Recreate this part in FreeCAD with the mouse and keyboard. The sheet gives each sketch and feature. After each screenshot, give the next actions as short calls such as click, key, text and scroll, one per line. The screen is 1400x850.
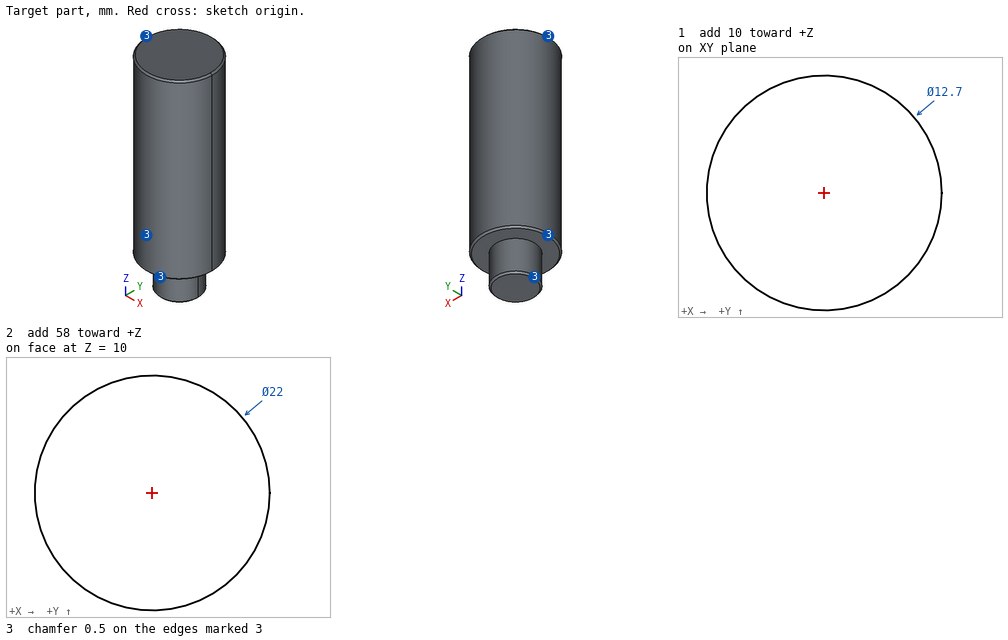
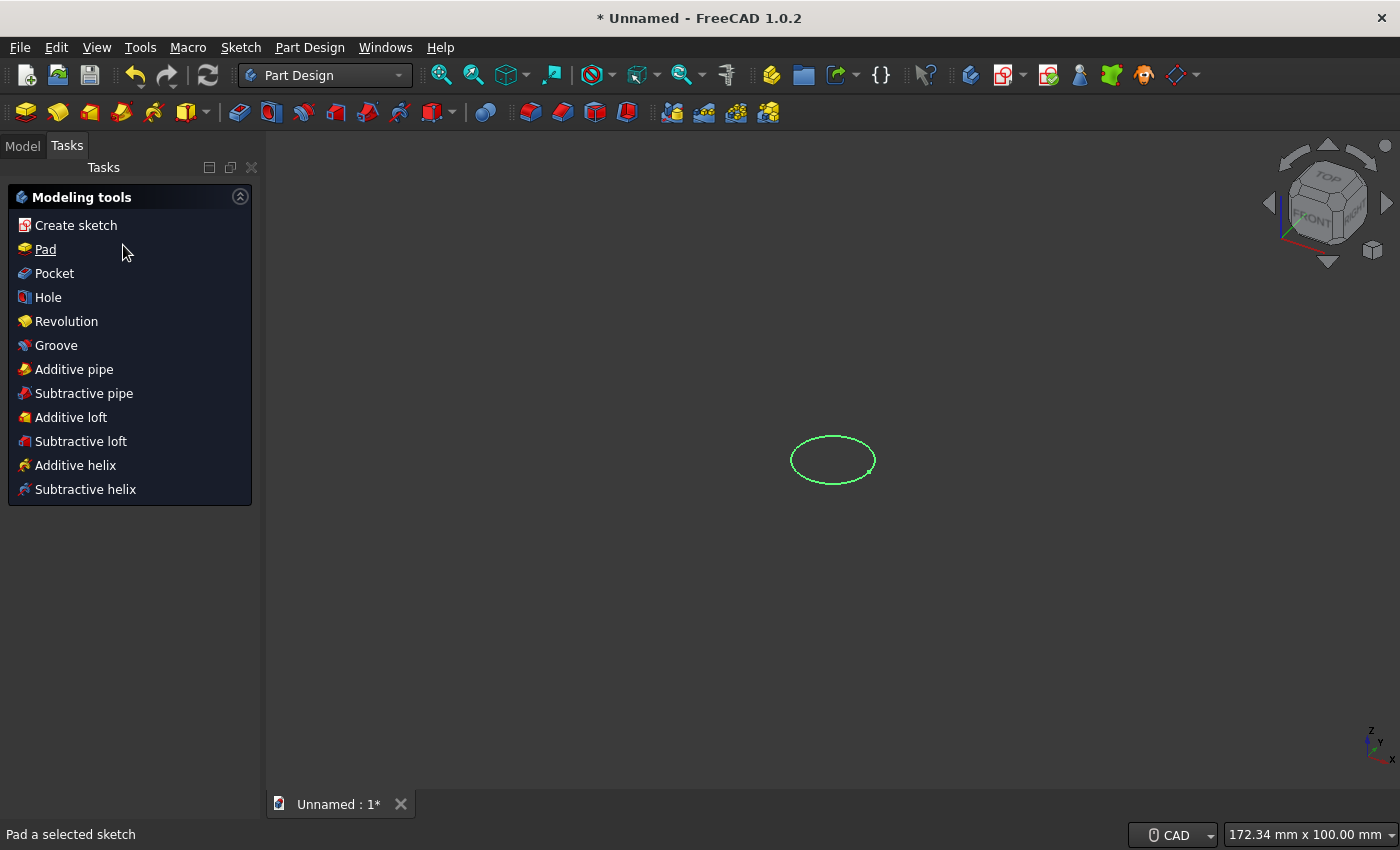
click(26, 112)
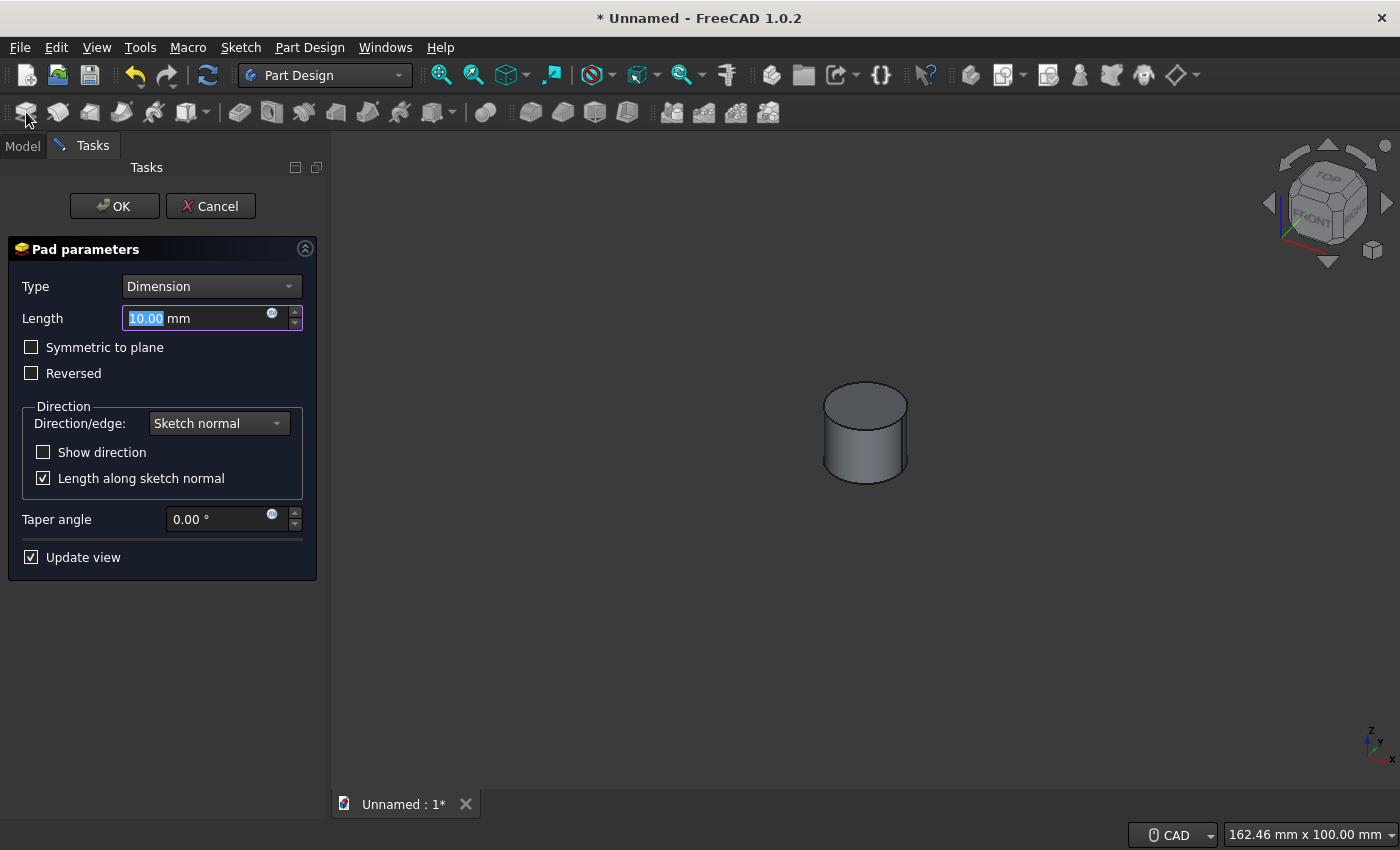
text(10)
key(Tab)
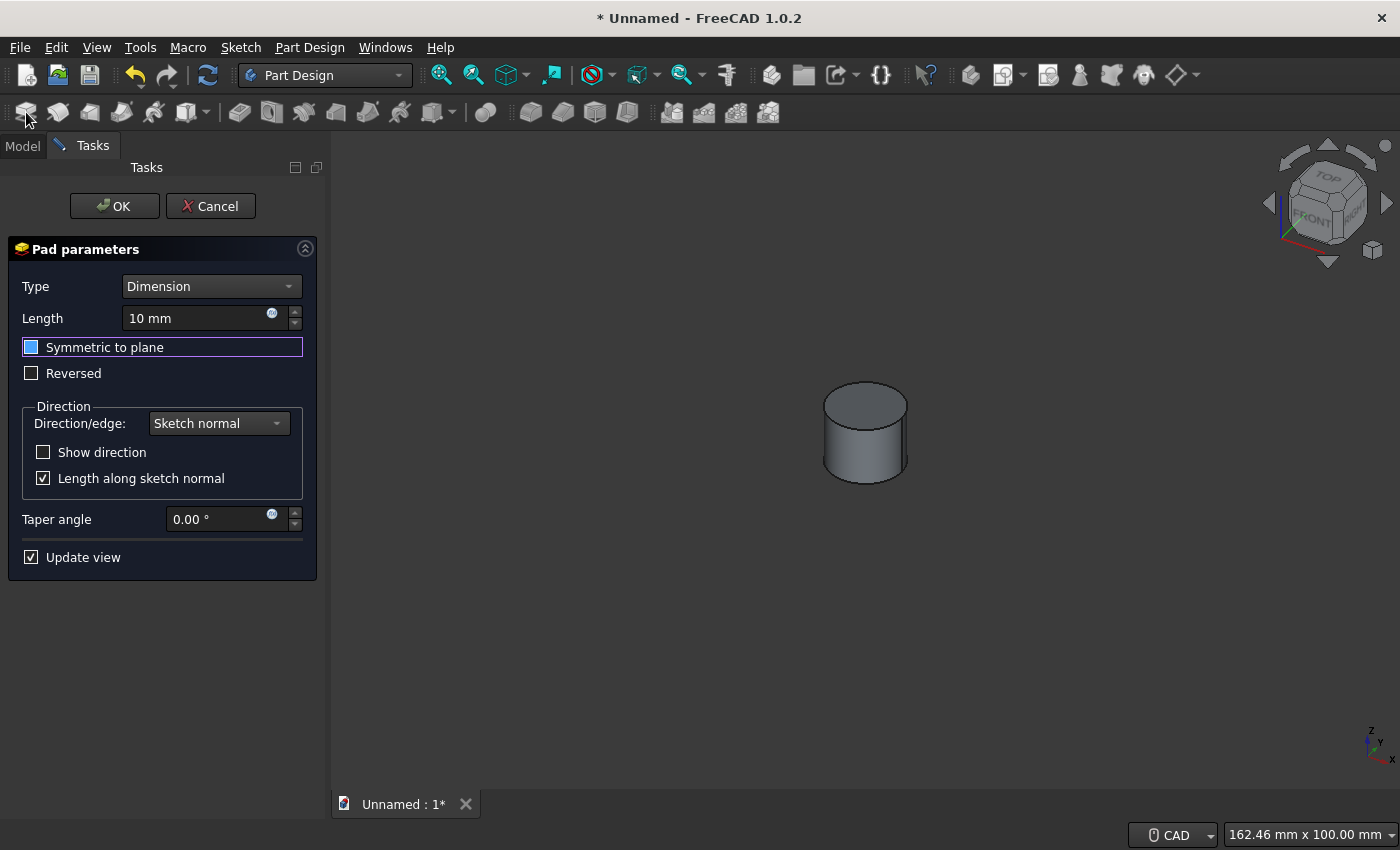
click(115, 206)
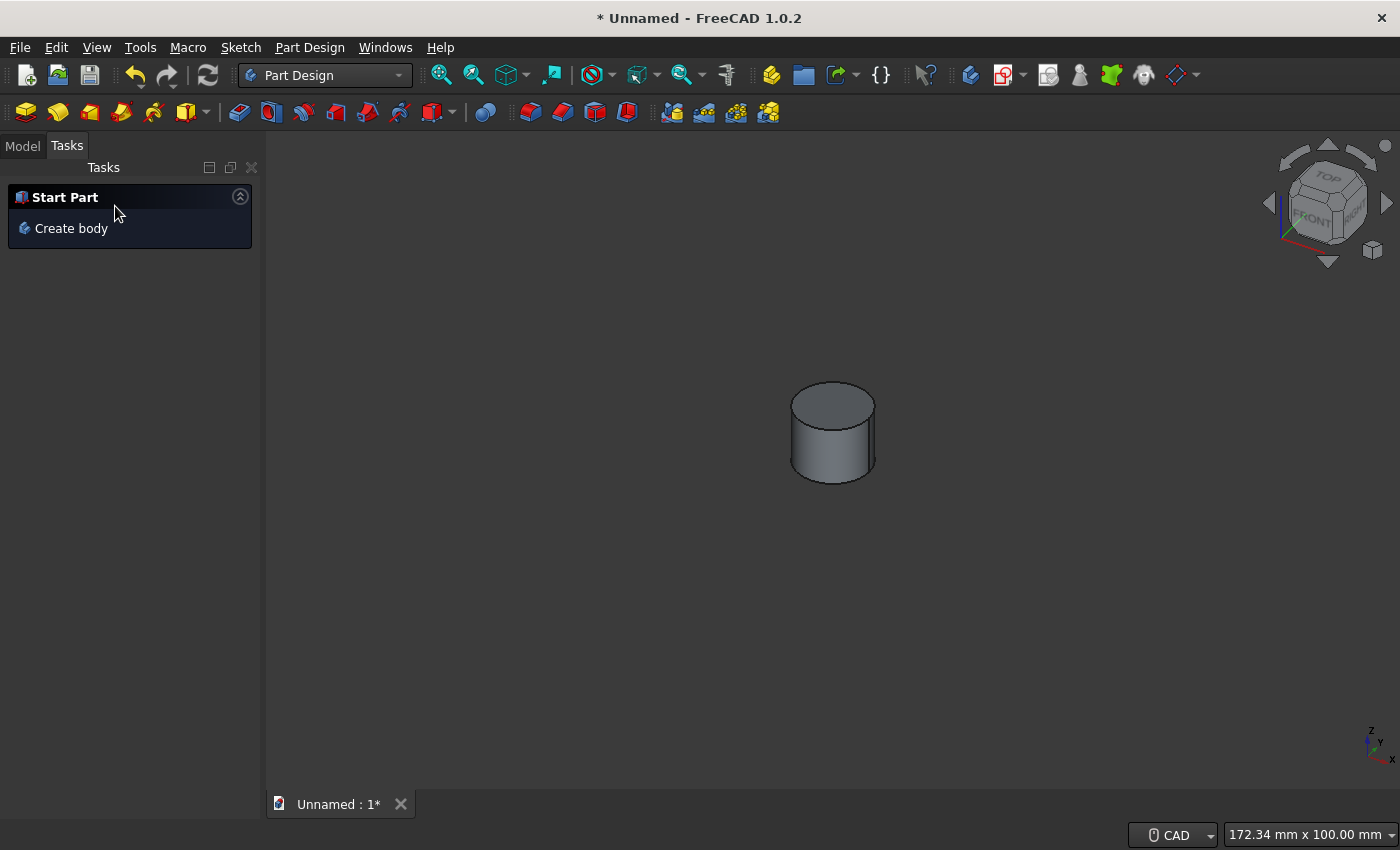
click(442, 76)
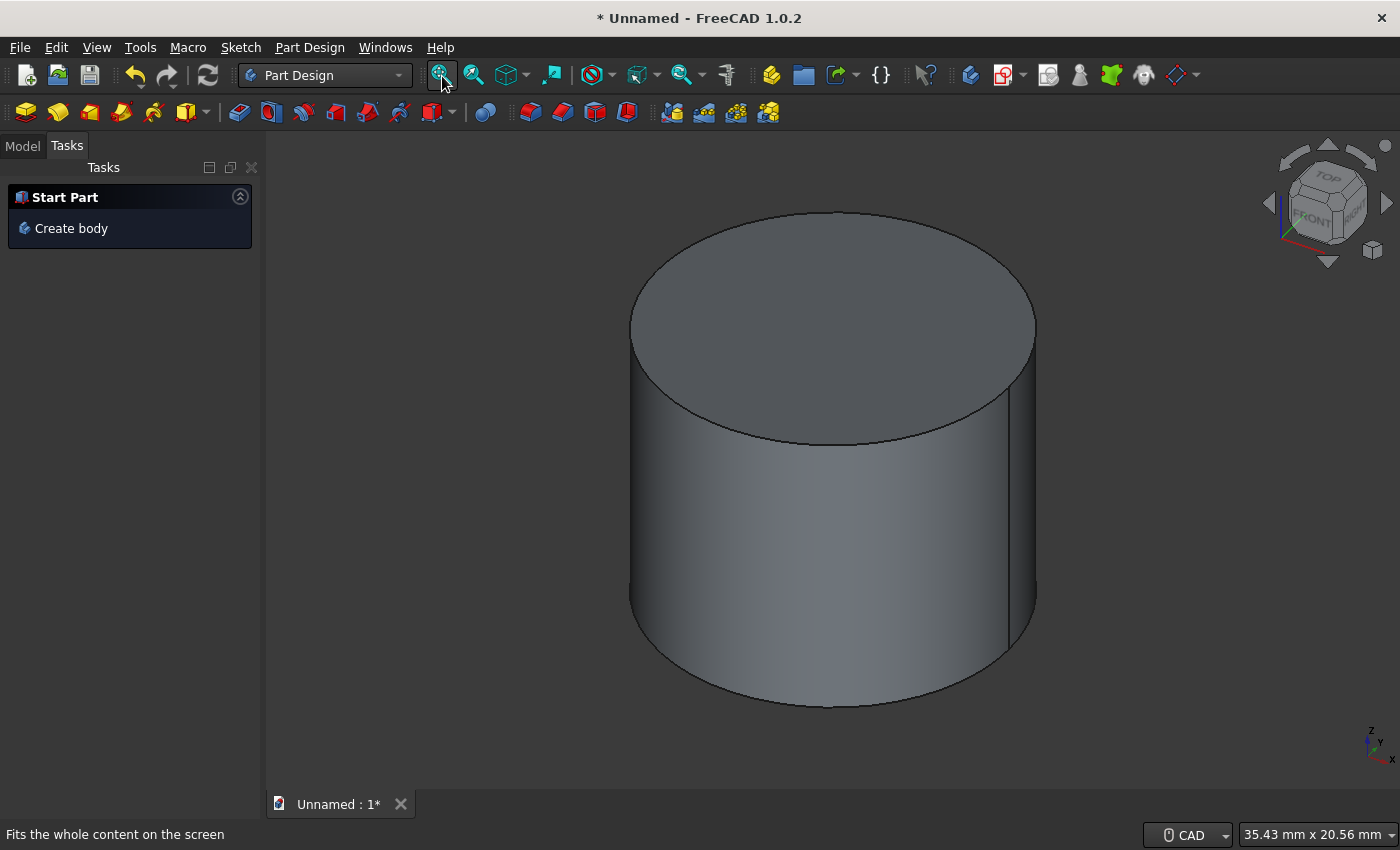
click(833, 328)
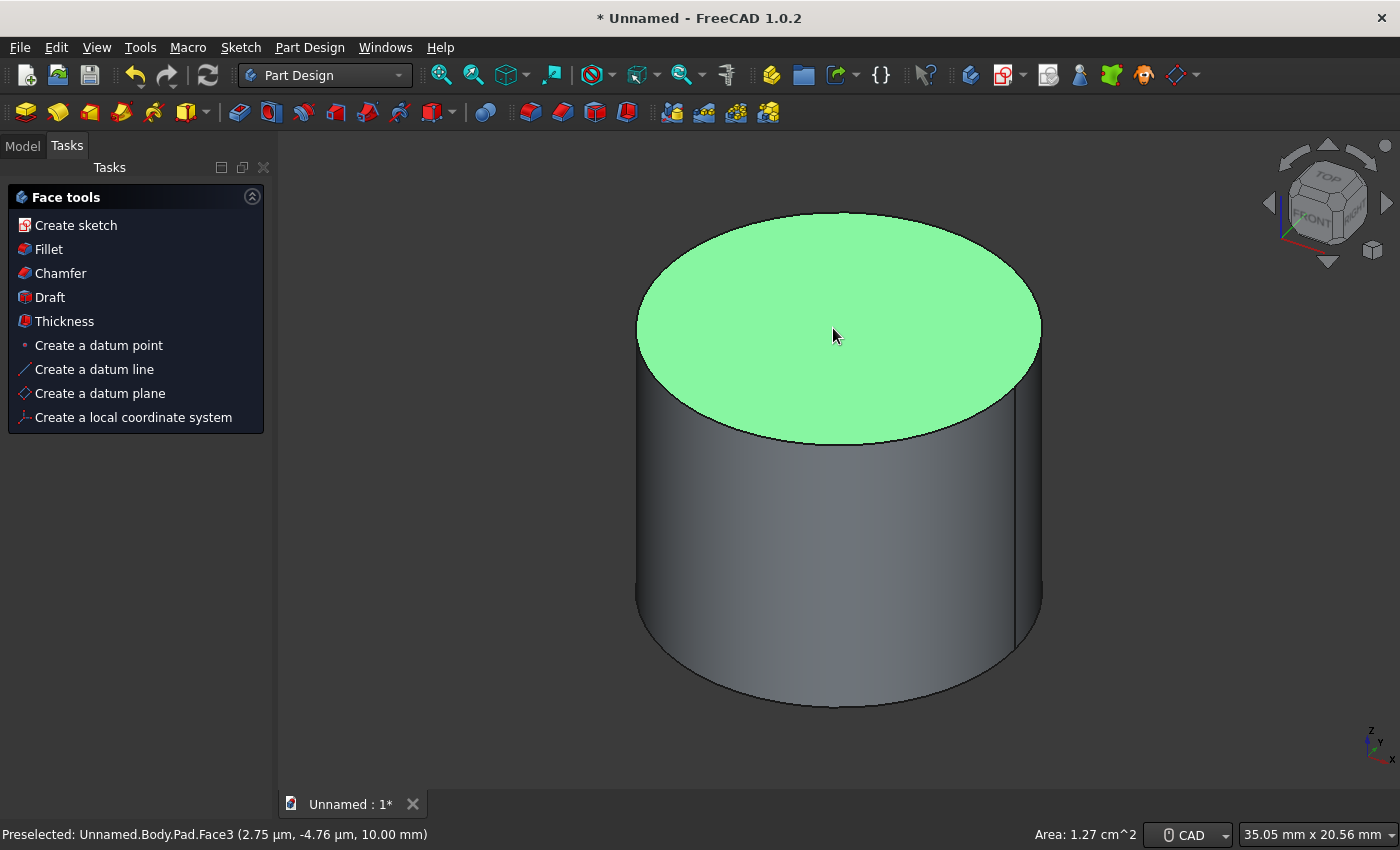
click(1004, 76)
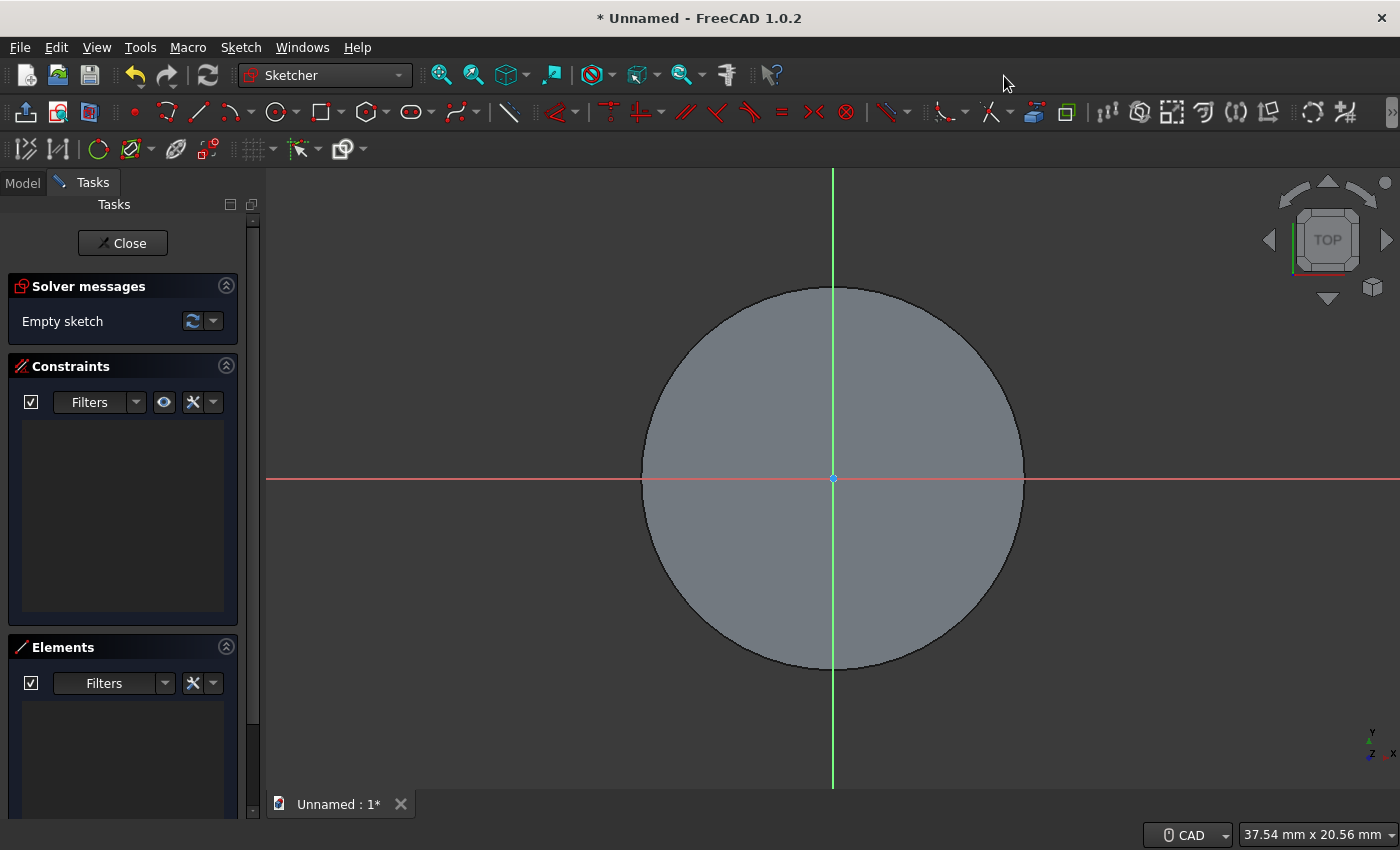
scroll(681, 478, down, 3)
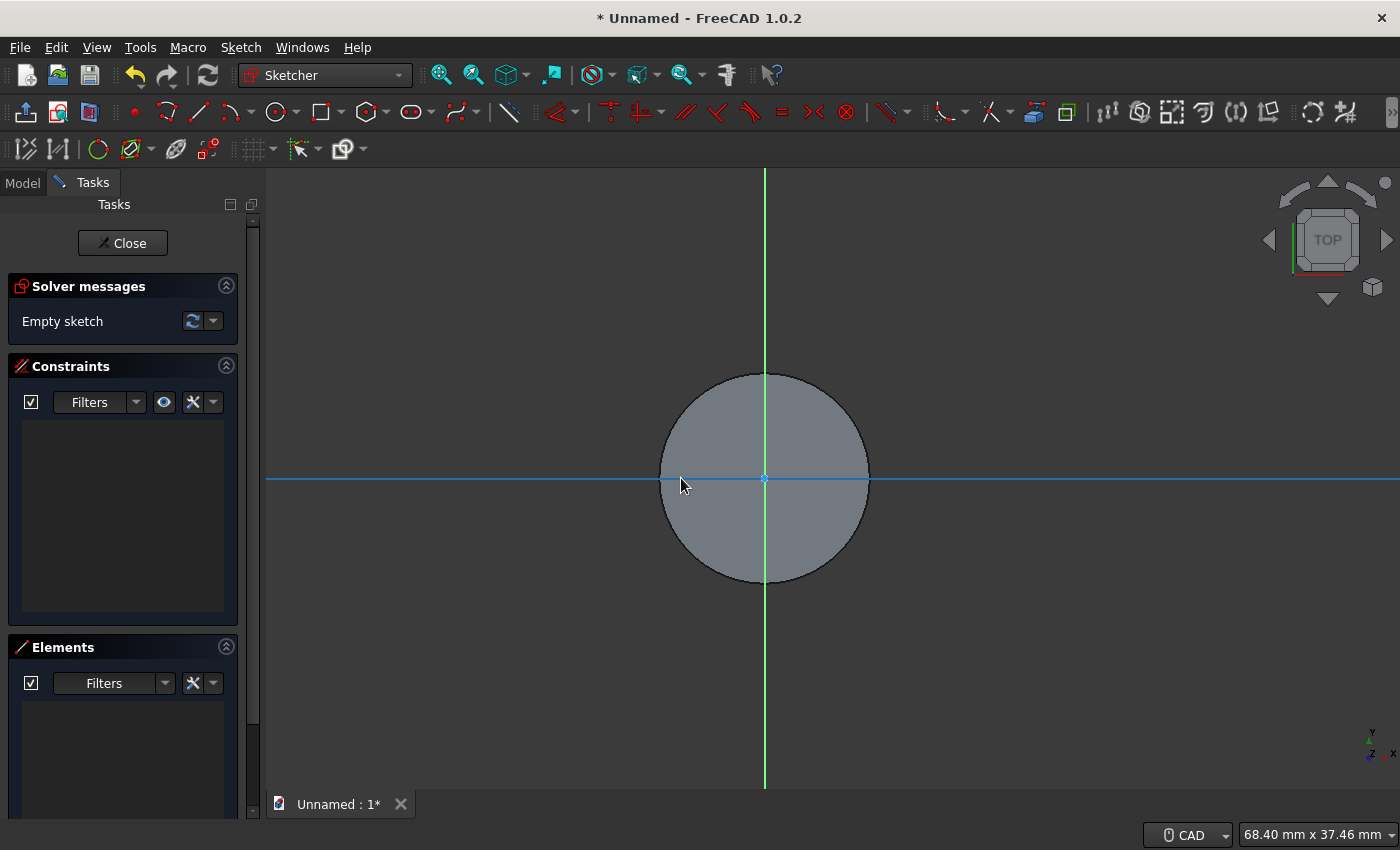
click(276, 112)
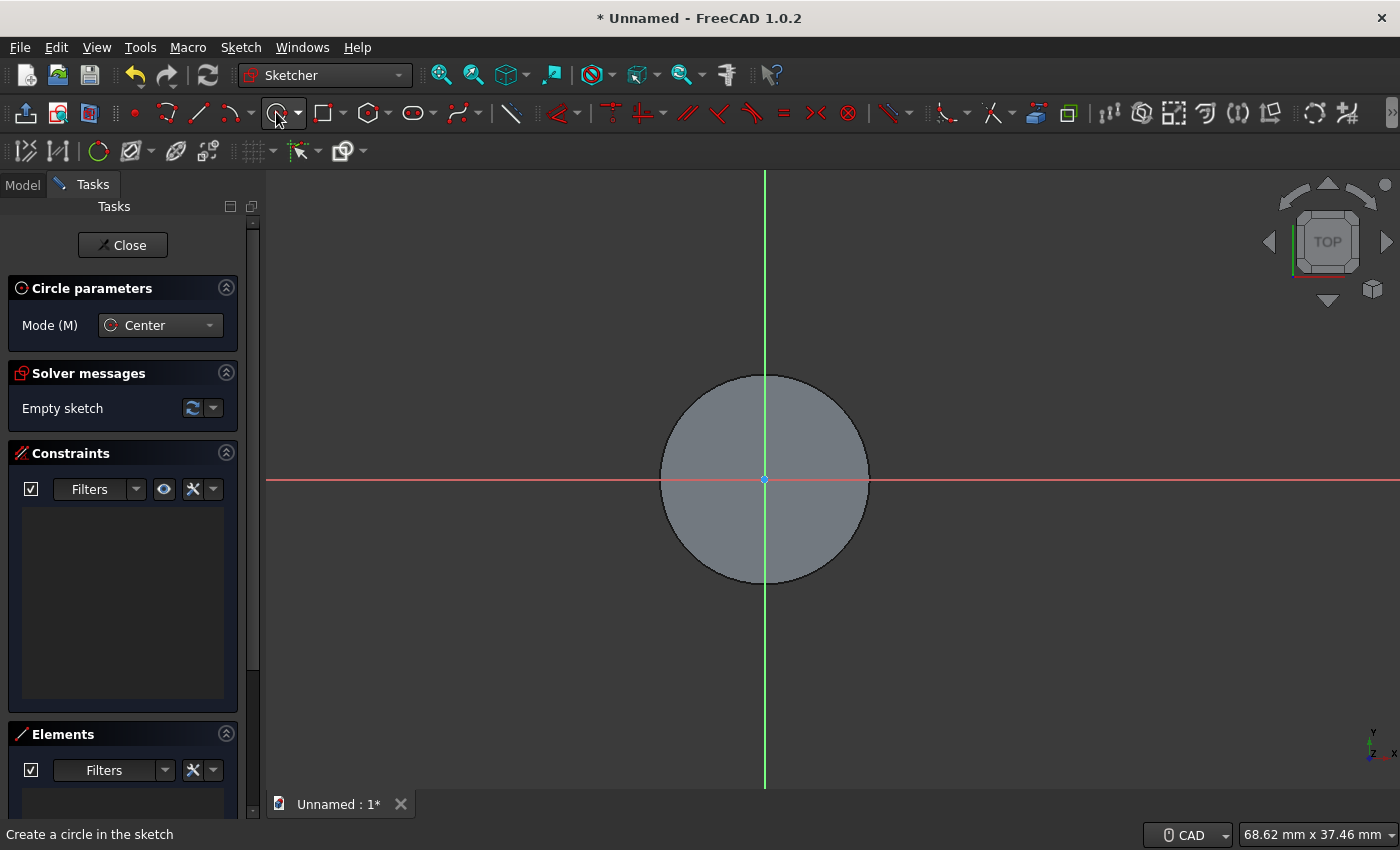
click(765, 480)
move(893, 351)